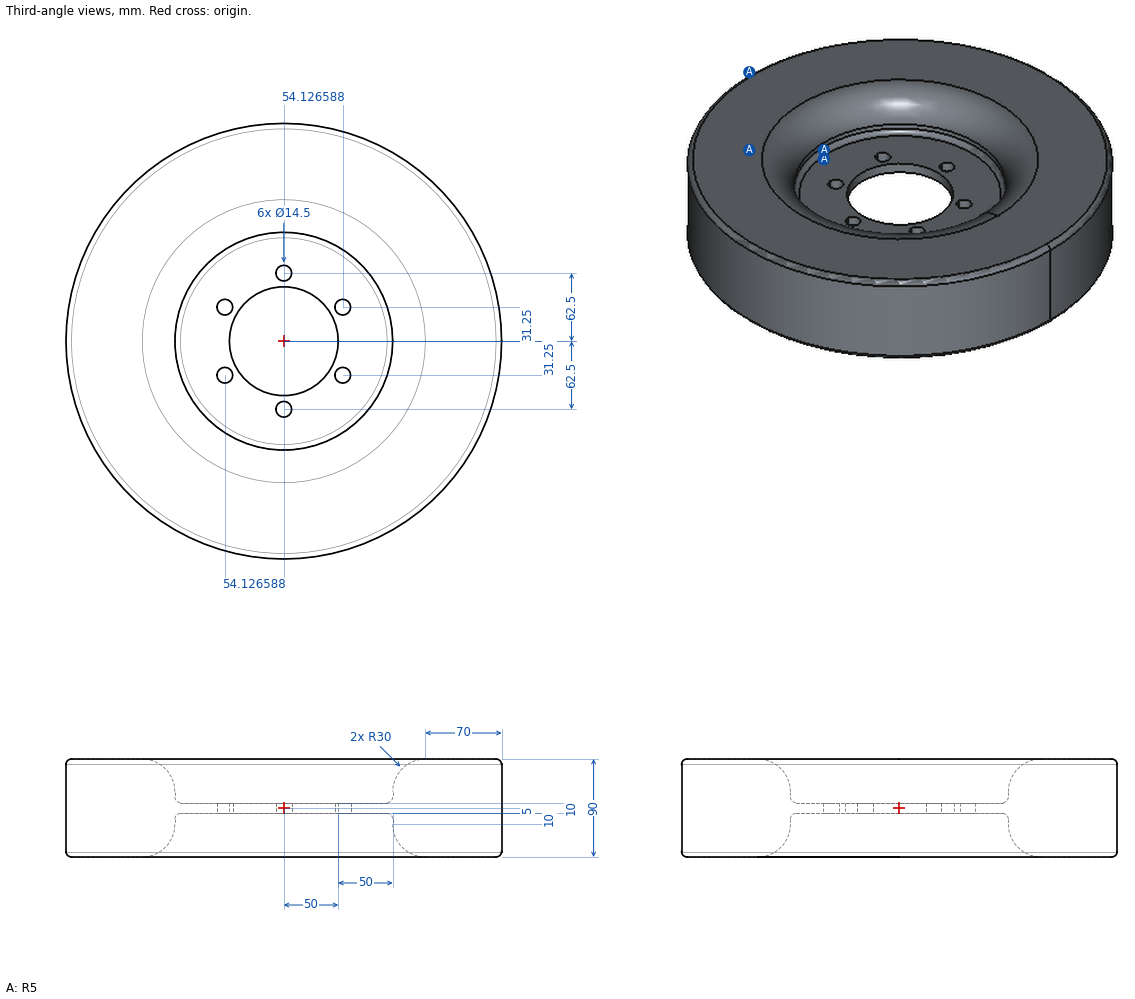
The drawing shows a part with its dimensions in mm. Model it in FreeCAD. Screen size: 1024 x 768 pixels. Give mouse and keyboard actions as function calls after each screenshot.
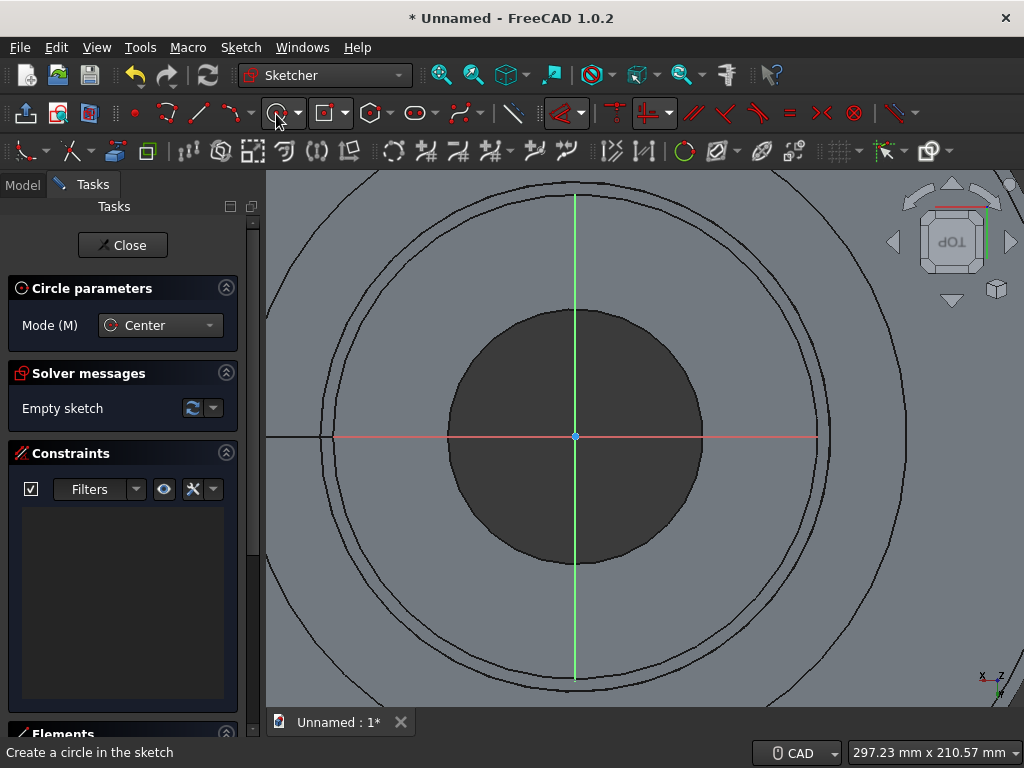
scroll(575, 596, up, 2)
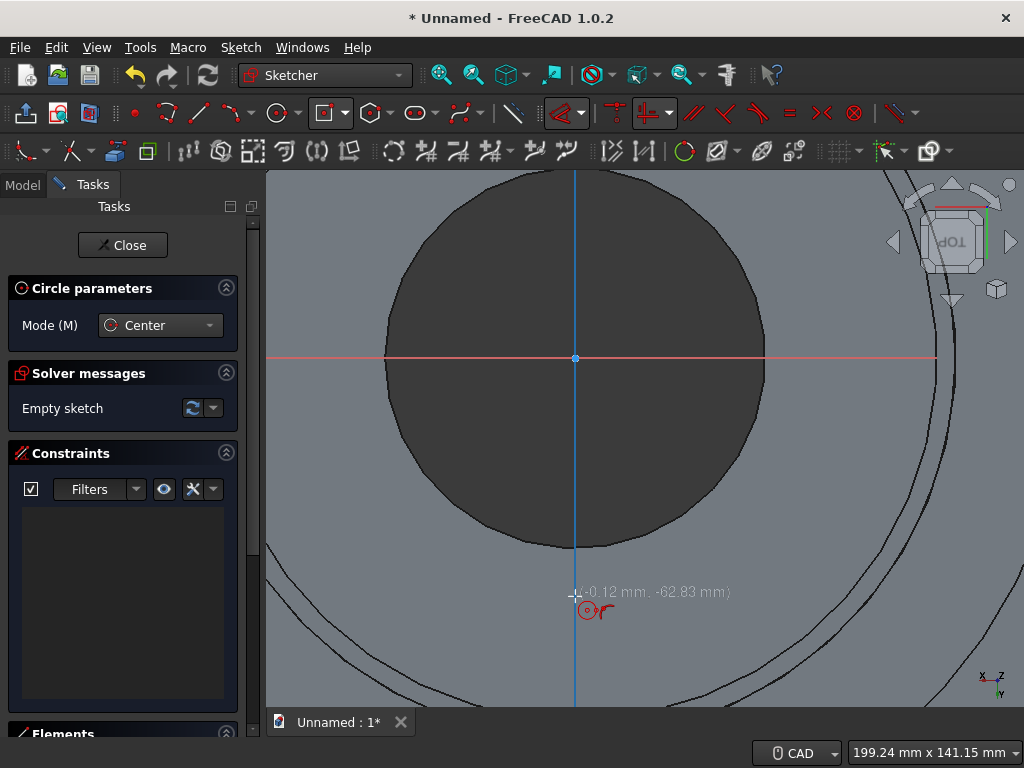
click(575, 596)
move(595, 576)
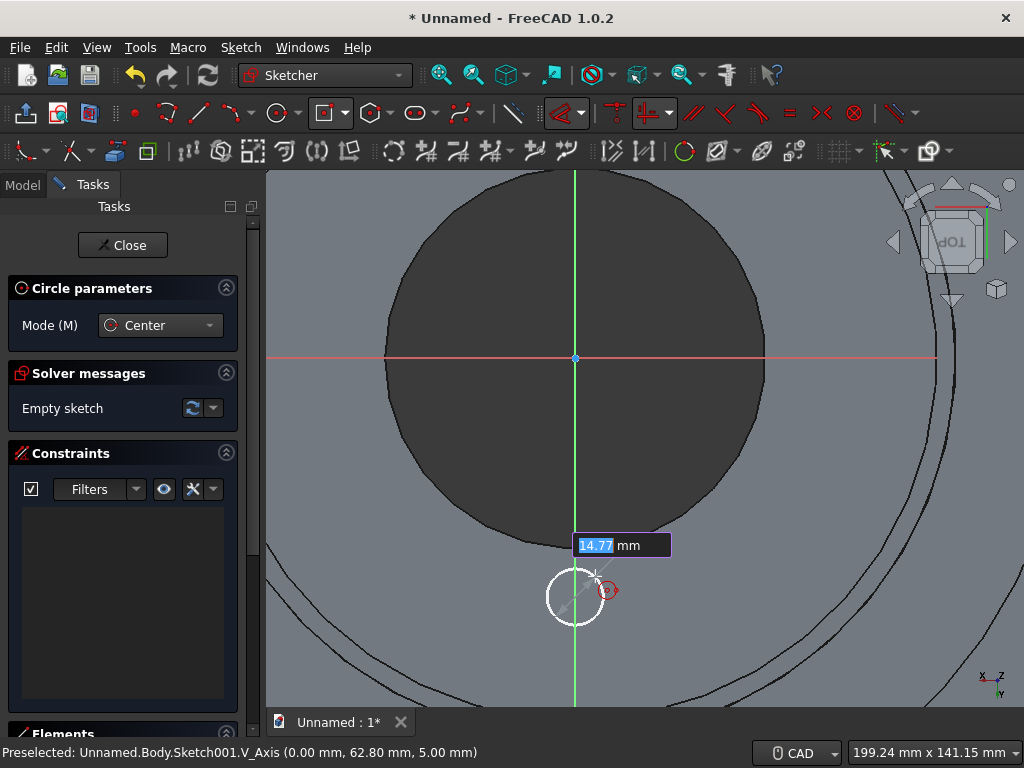
text(14.5)
key(Return)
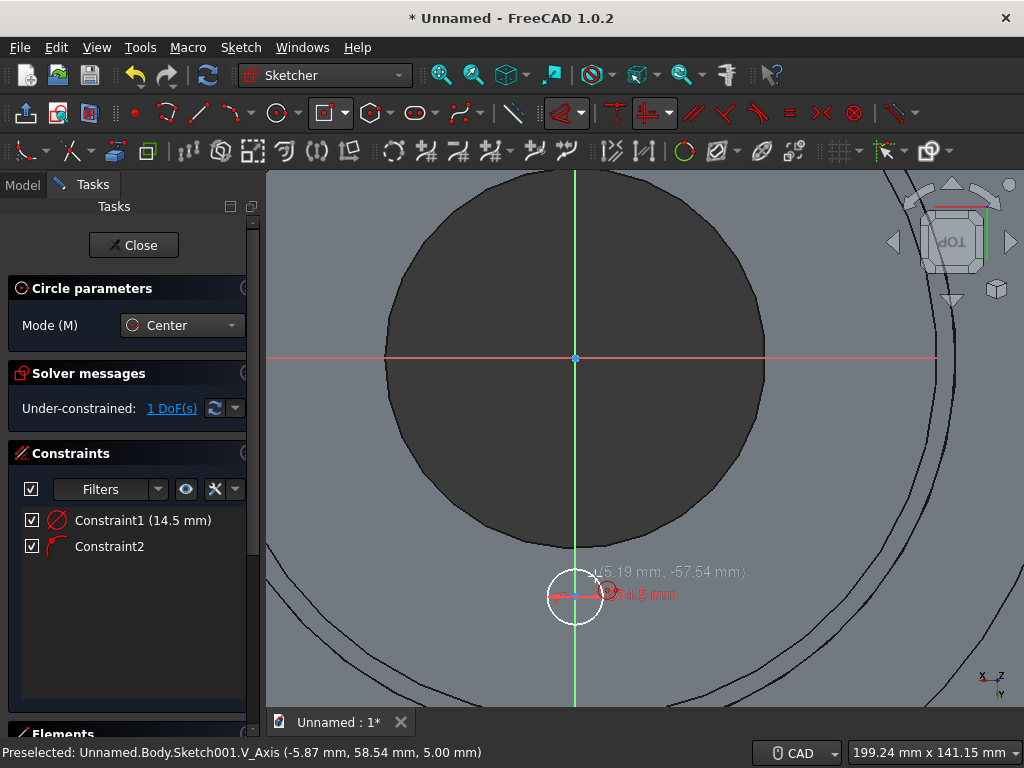
click(369, 477)
move(389, 457)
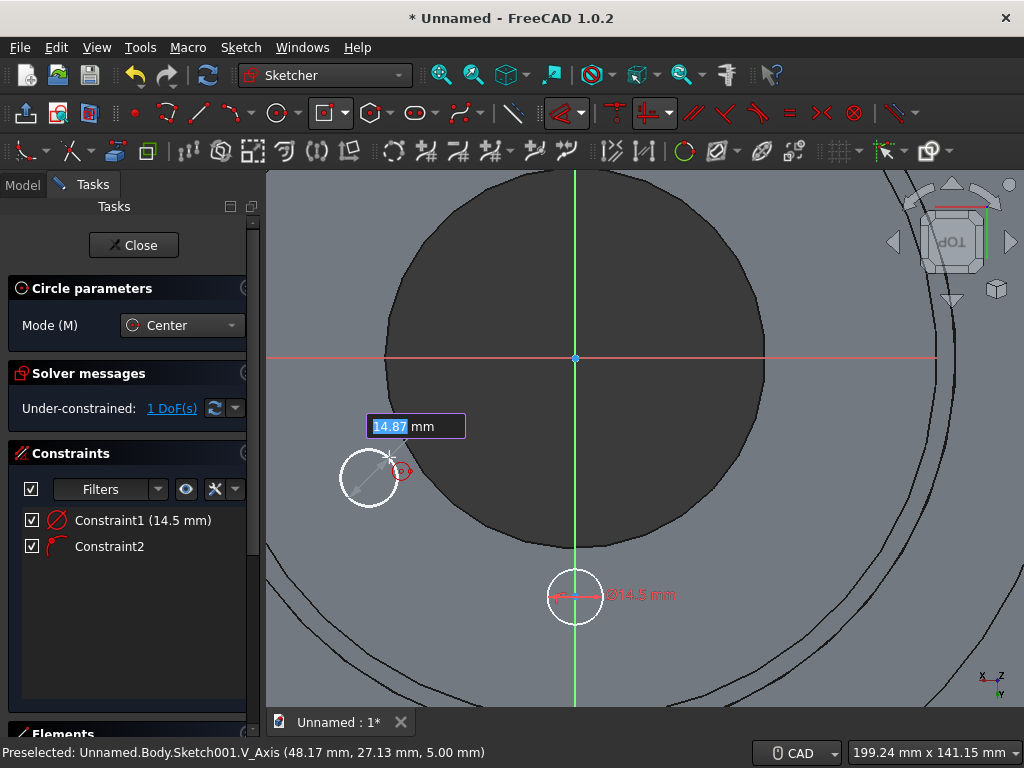
text(14.5)
key(Return)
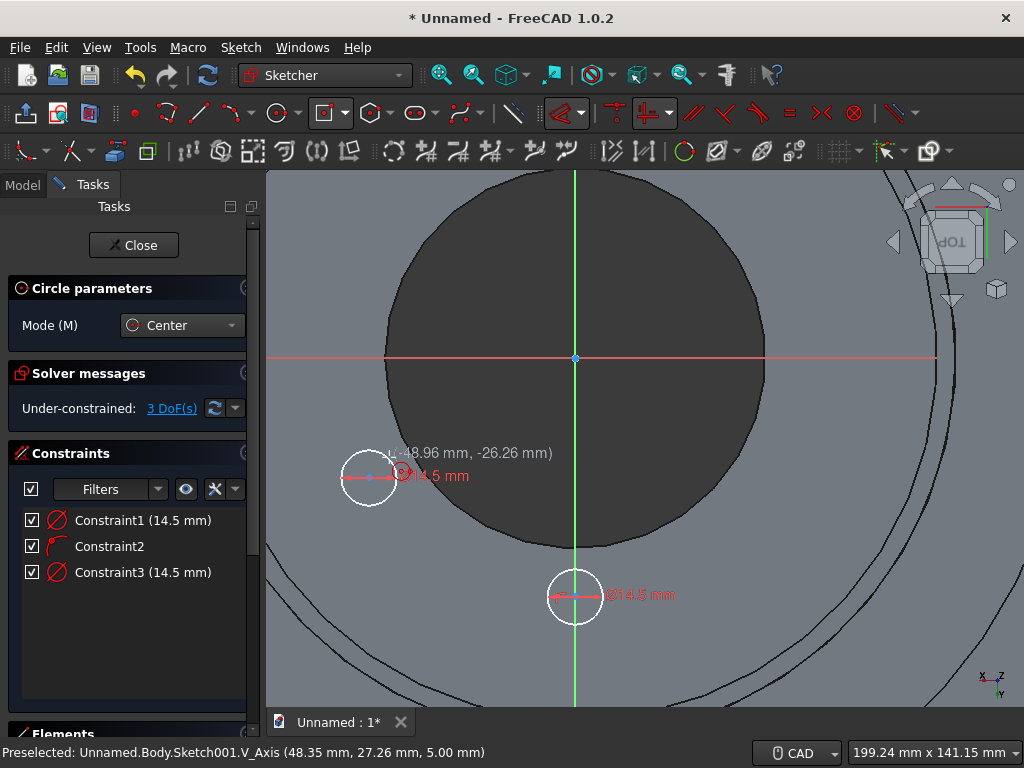
click(369, 239)
move(389, 220)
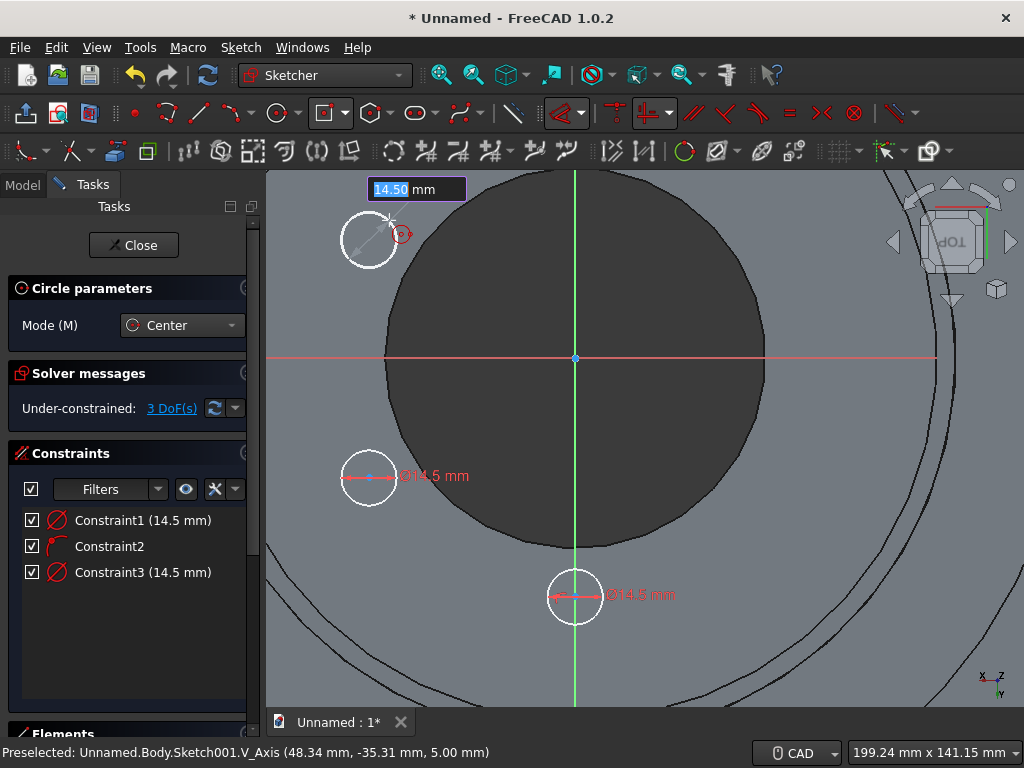
text(14.5)
key(Return)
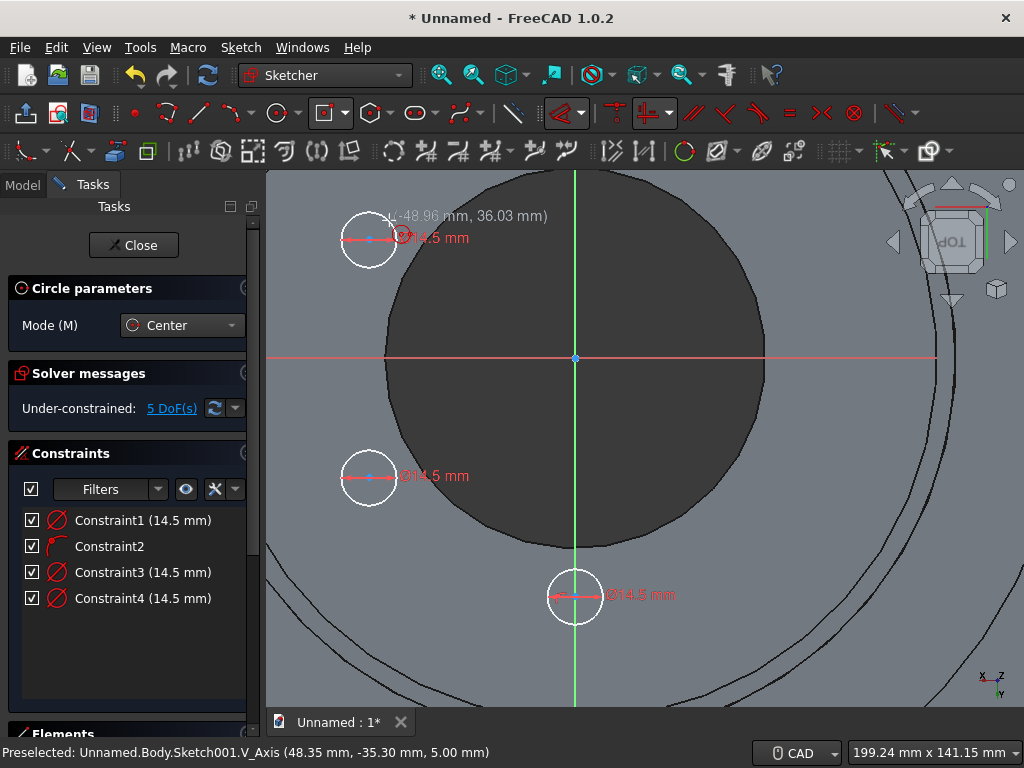
scroll(579, 602, down, 2)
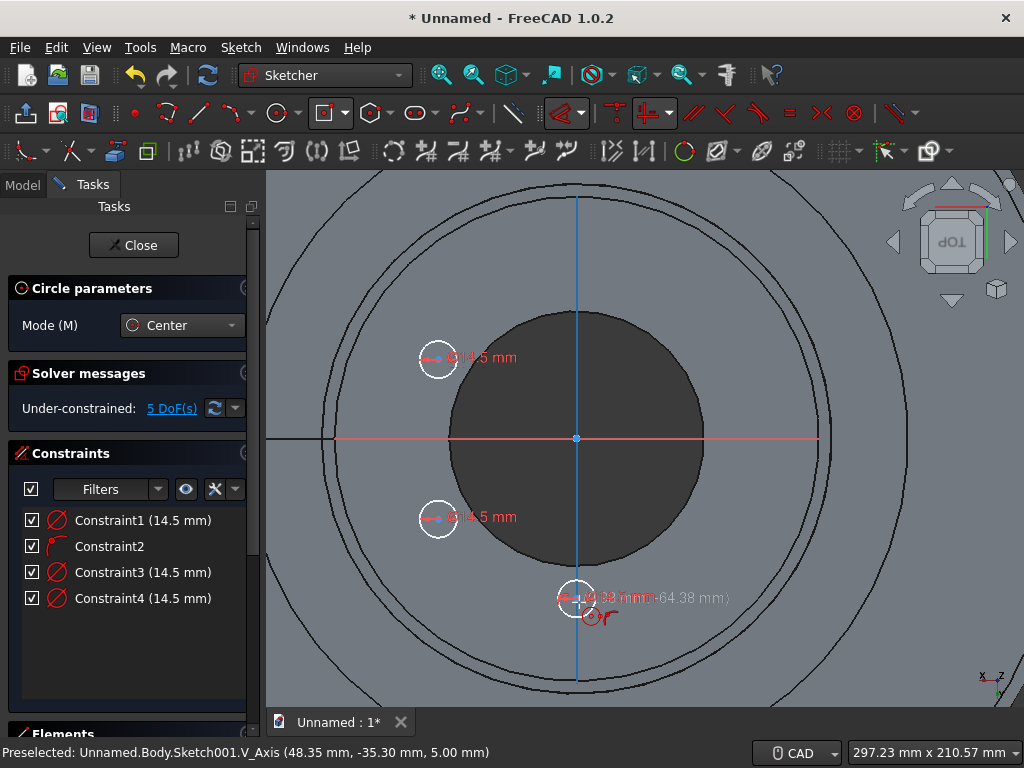
scroll(577, 279, up, 2)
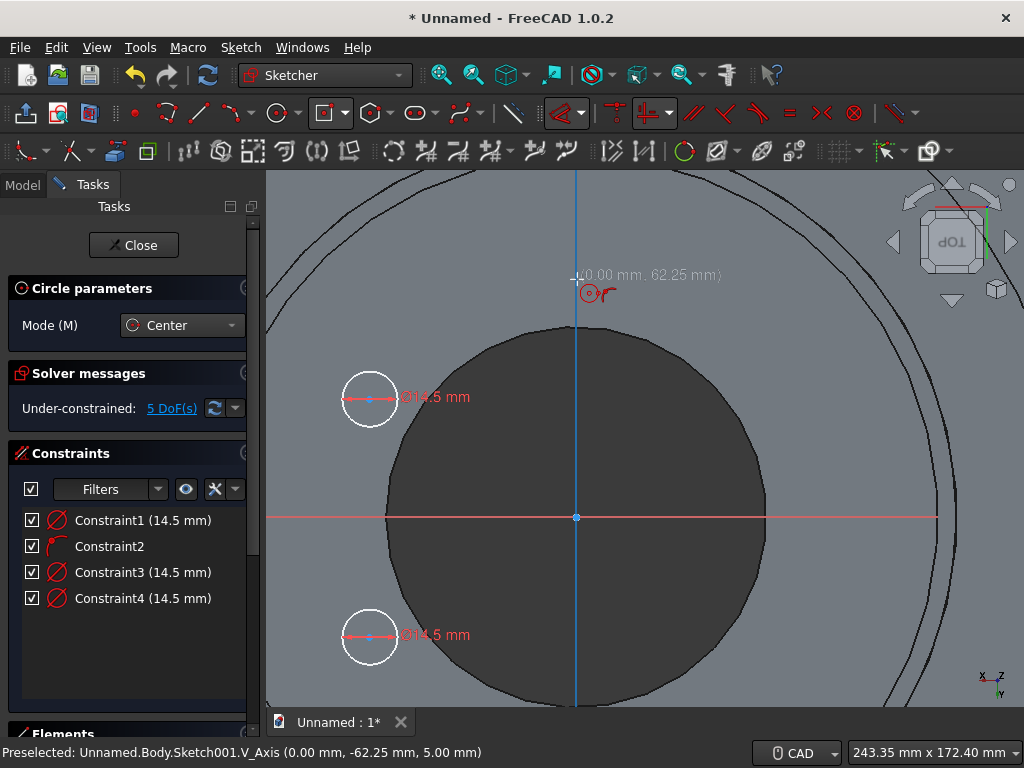
click(576, 279)
move(596, 260)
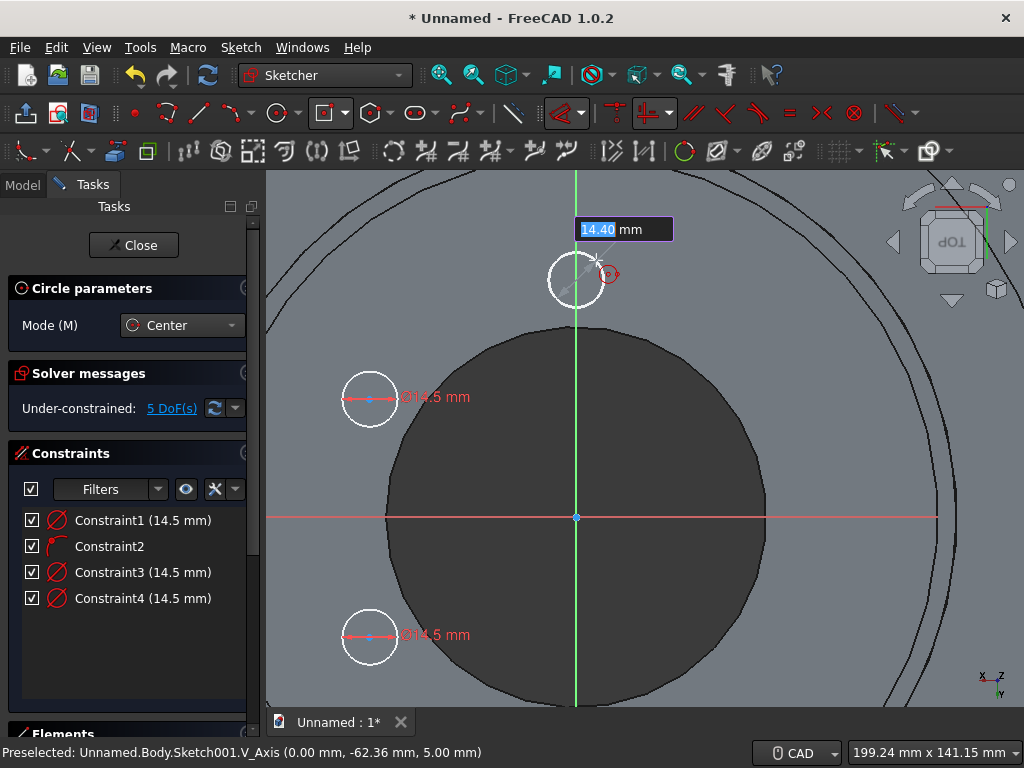
text(14.5)
key(Return)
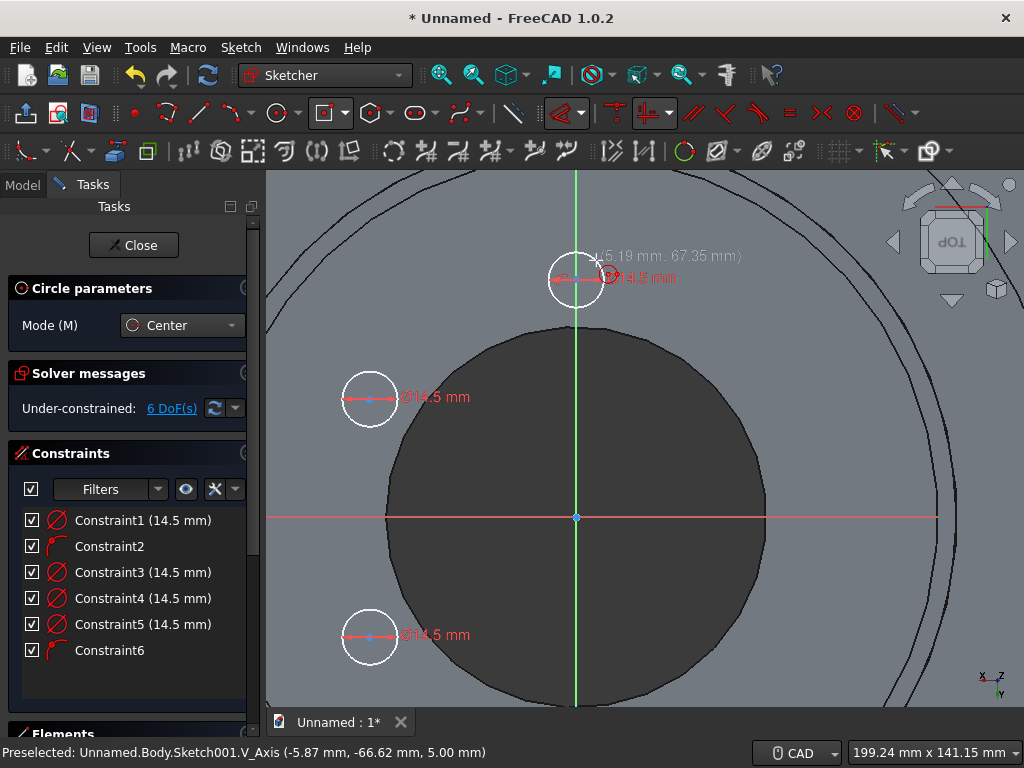
click(782, 398)
move(802, 379)